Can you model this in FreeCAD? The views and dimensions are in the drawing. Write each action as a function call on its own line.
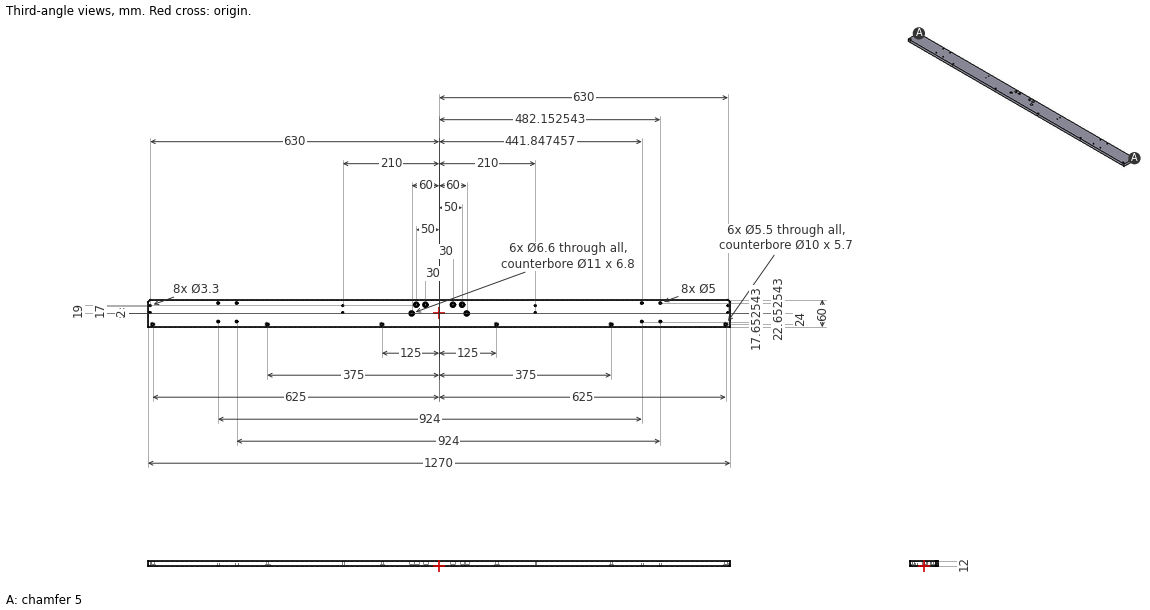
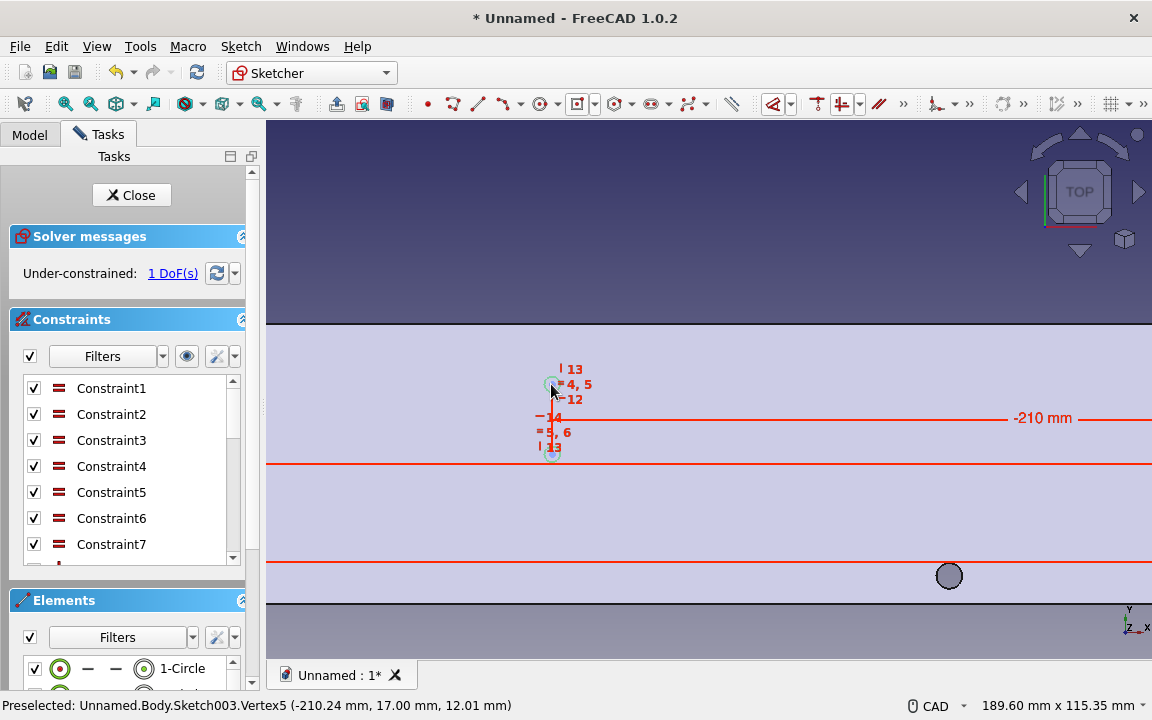
scroll(551, 386, down, 12)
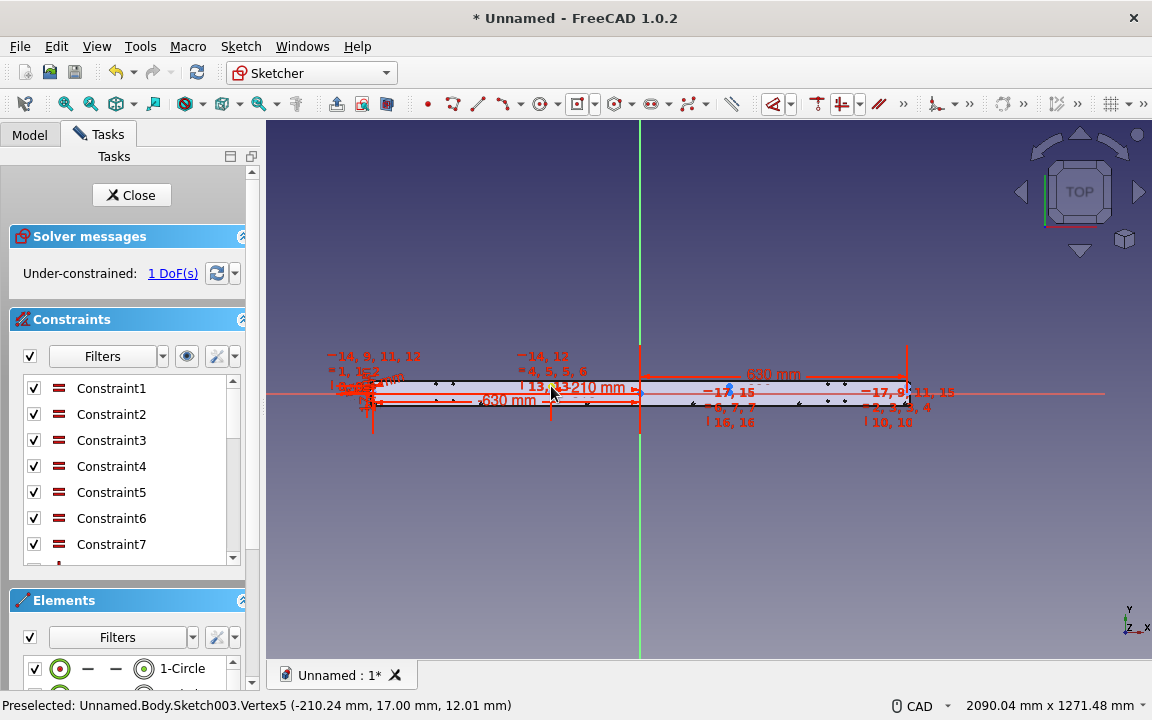
scroll(729, 393, up, 4)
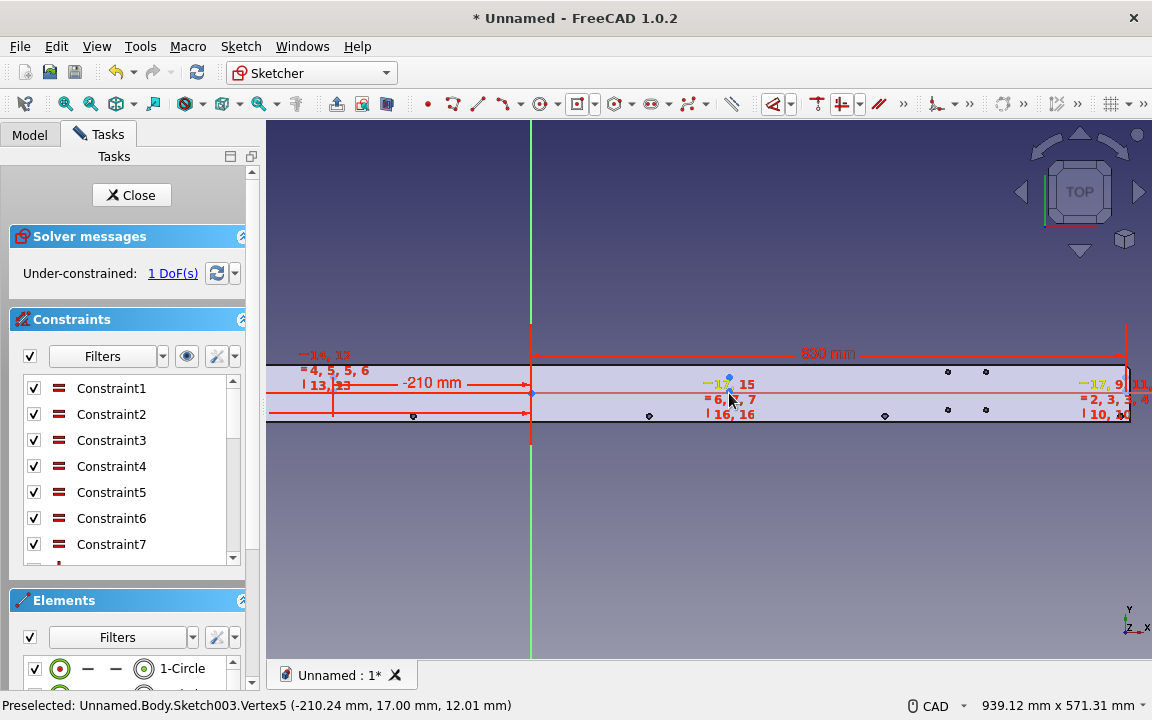
scroll(729, 392, up, 4)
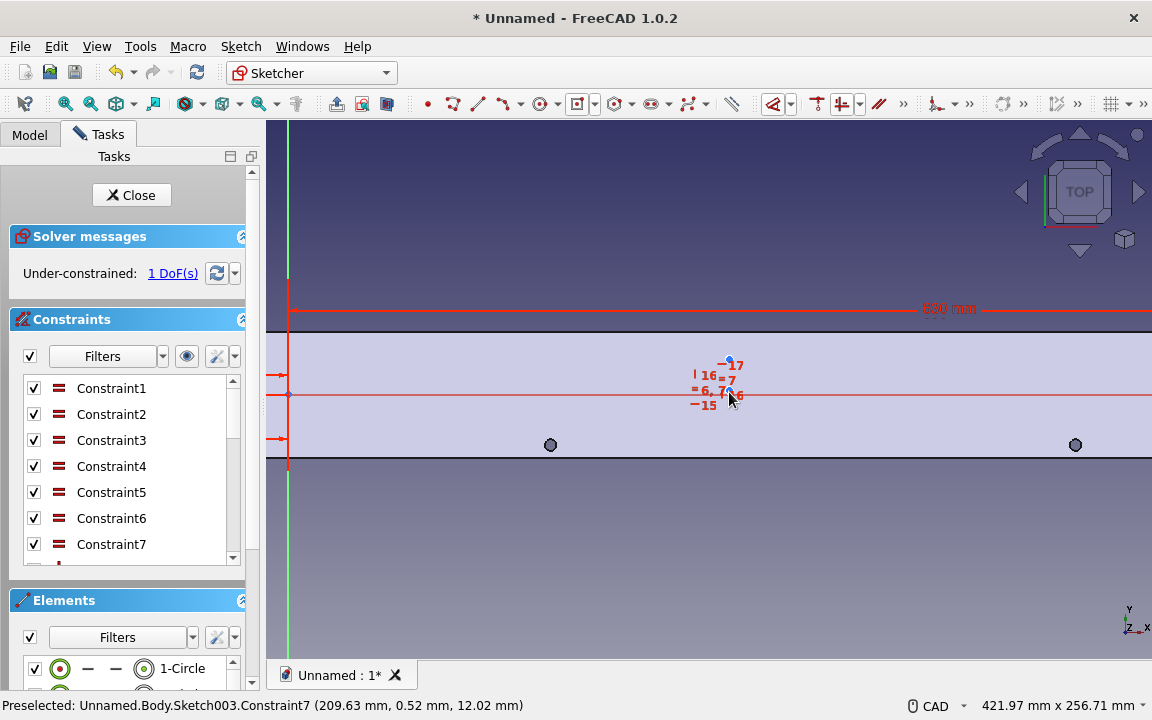
scroll(729, 391, up, 4)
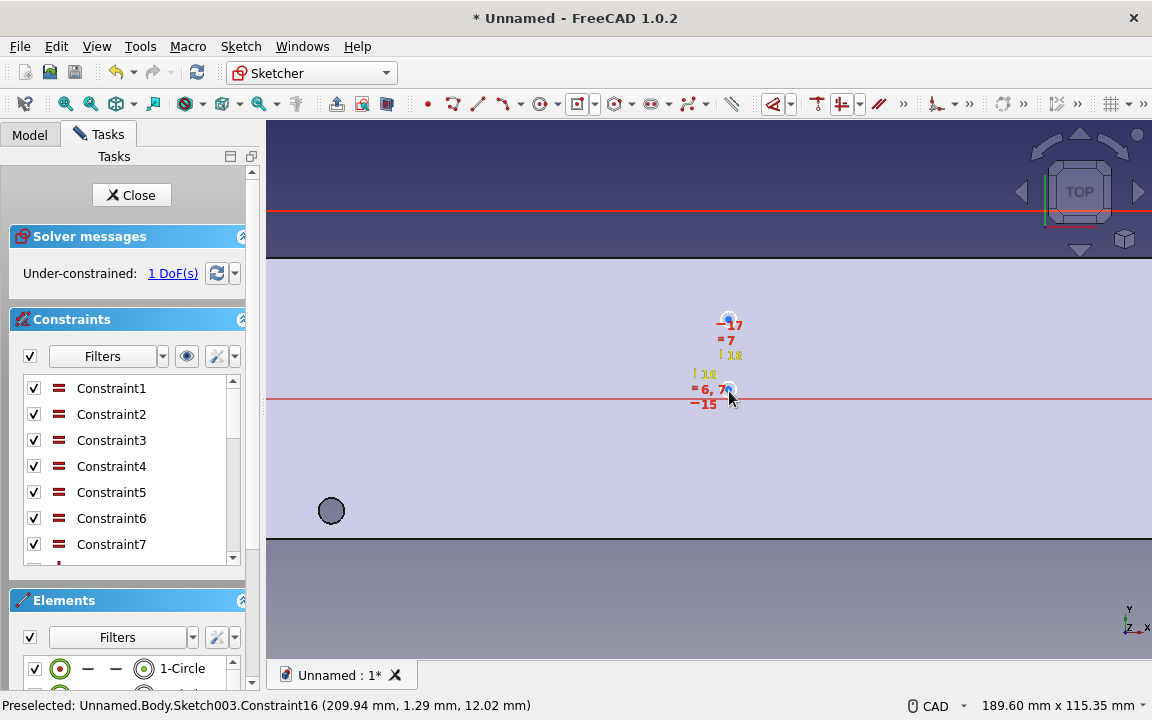
click(729, 389)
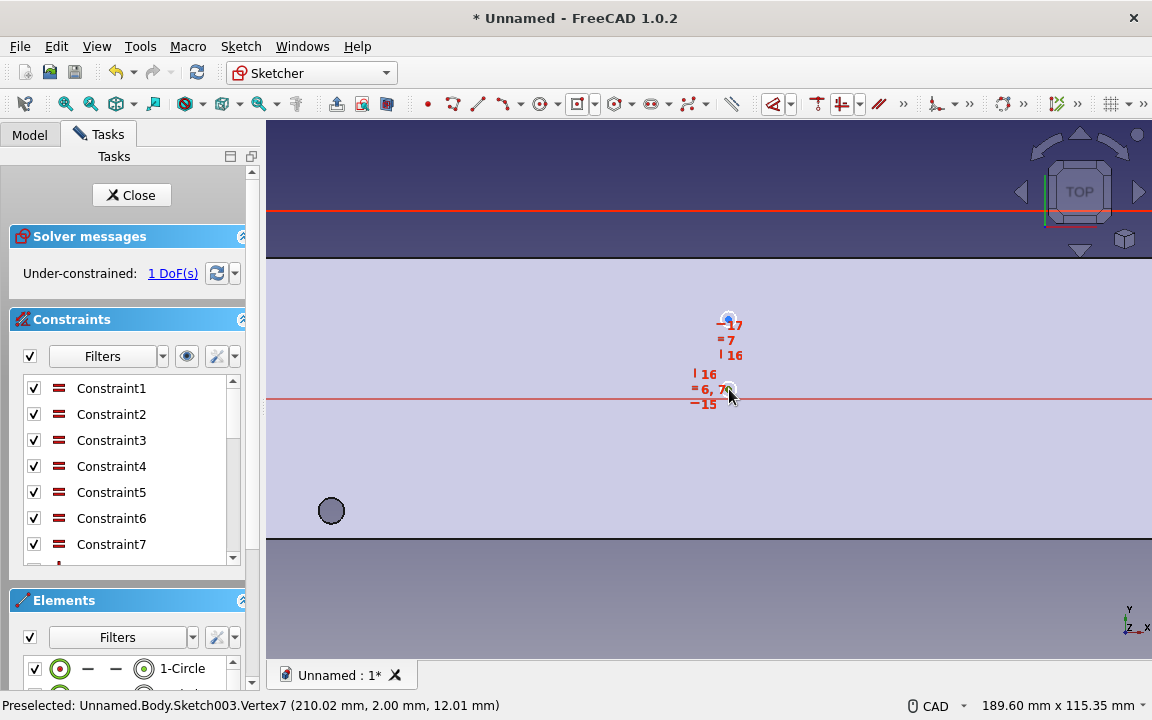
key(l)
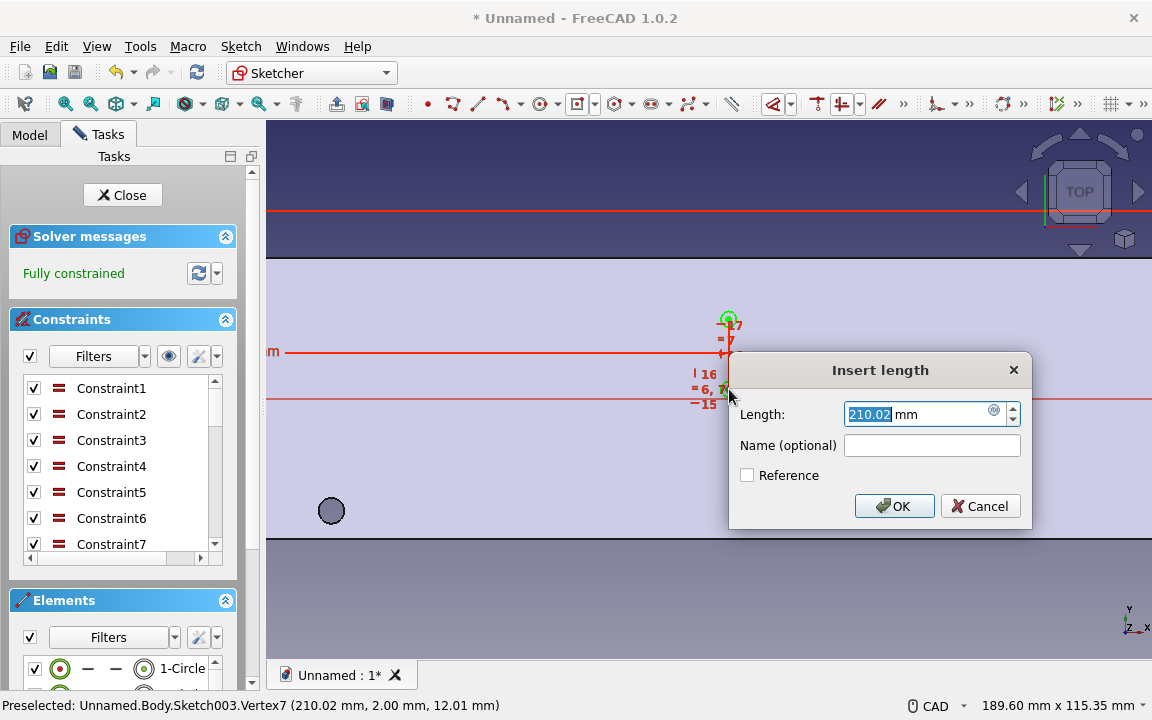
text(210)
key(Return)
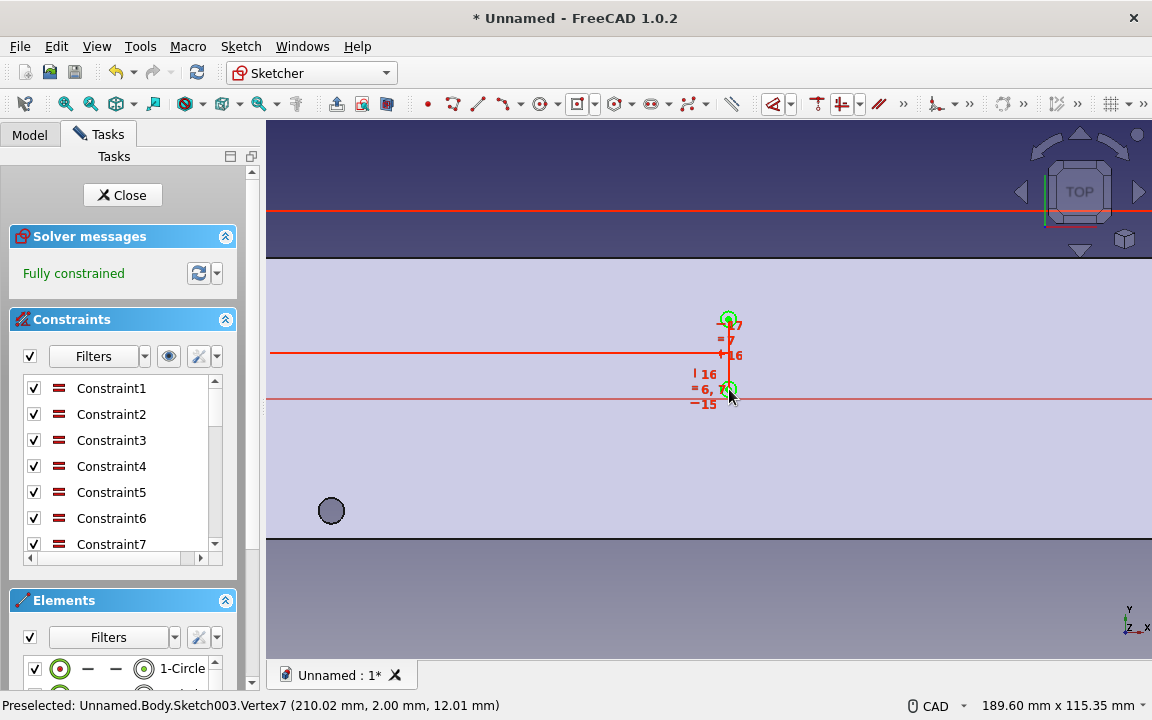
click(123, 195)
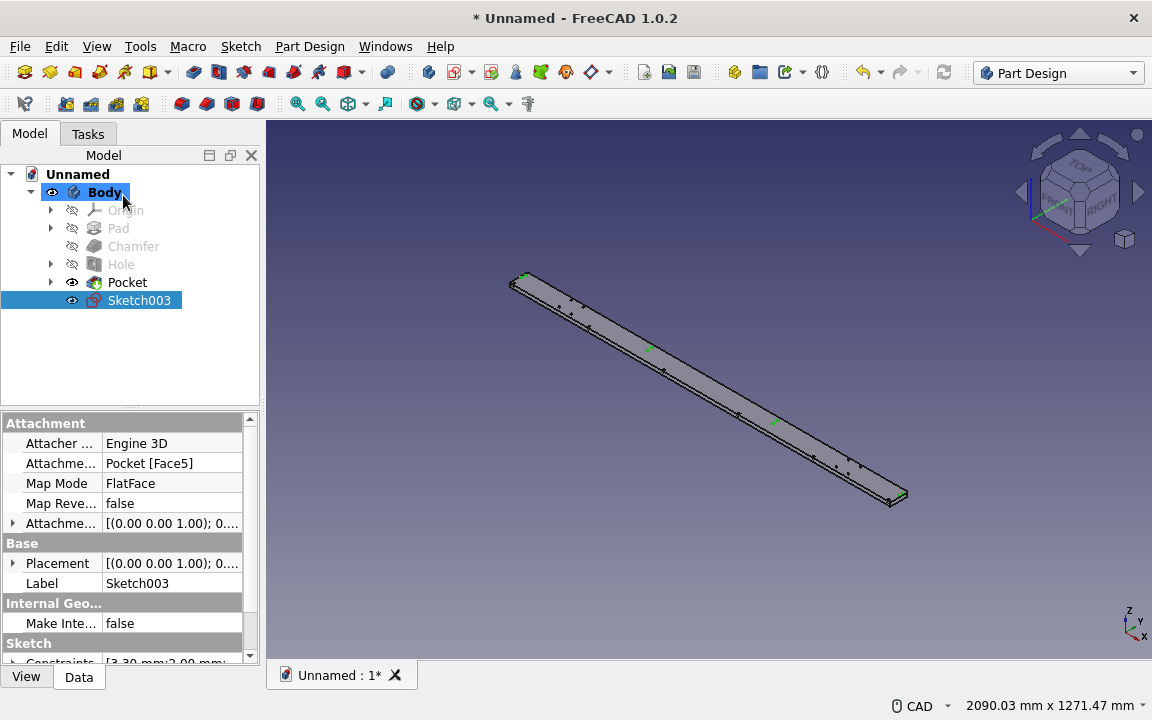
click(194, 72)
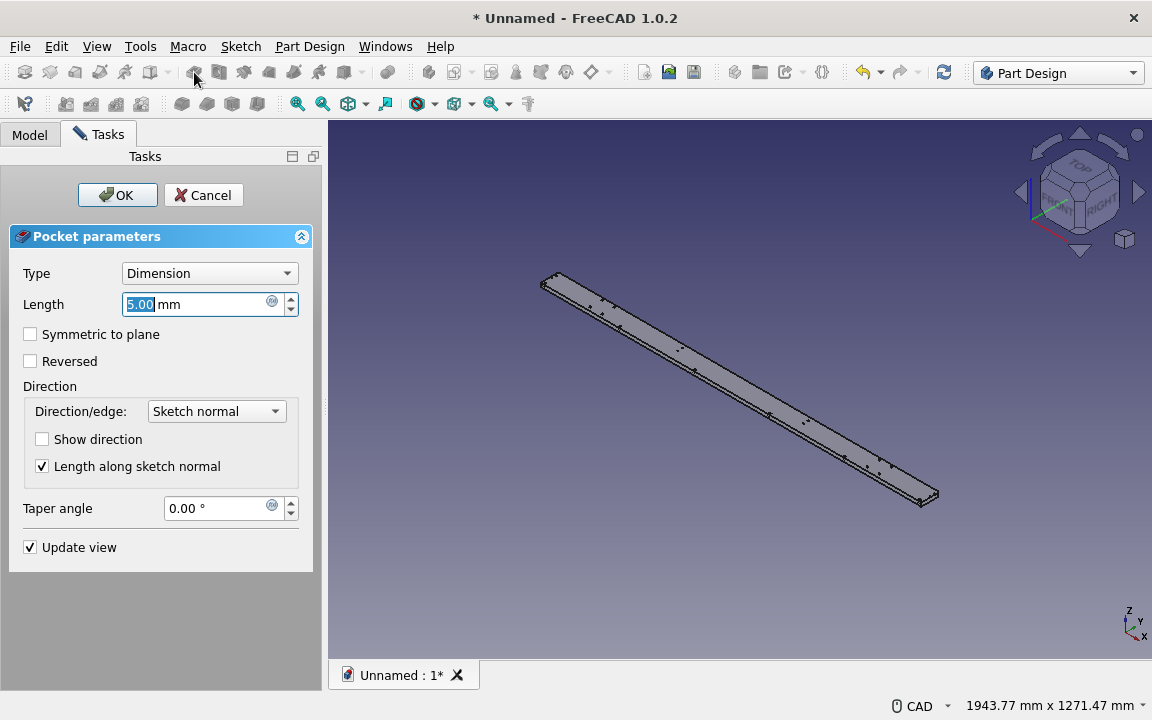
click(210, 274)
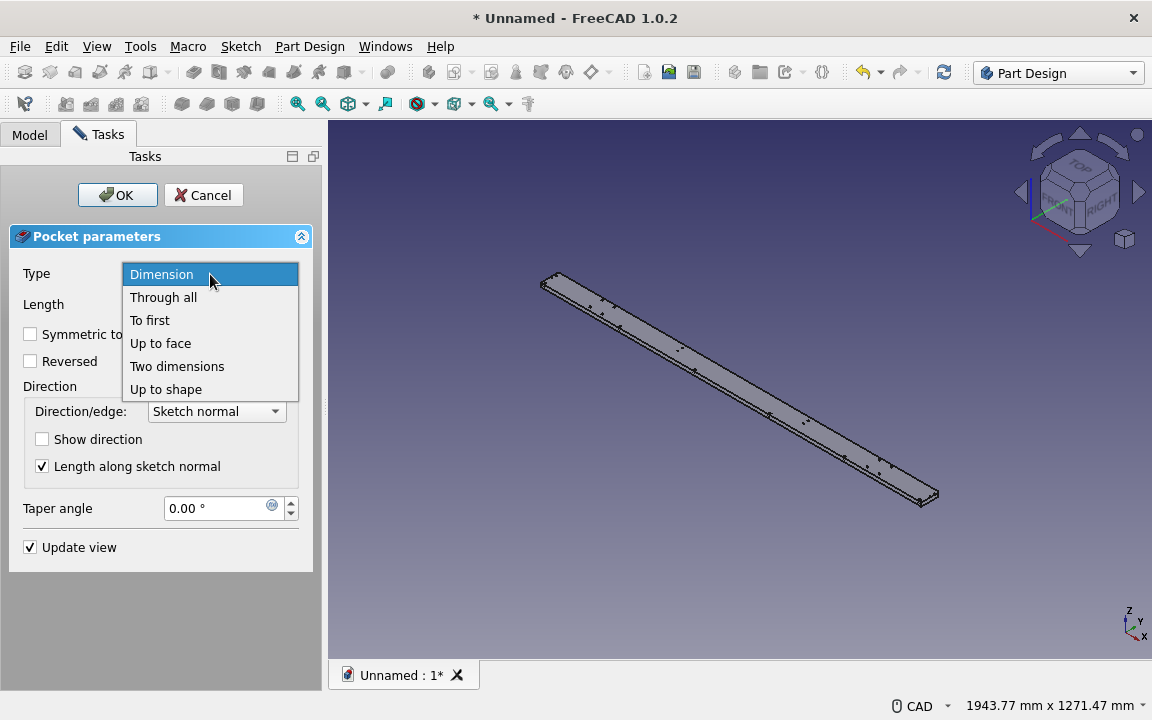
click(208, 298)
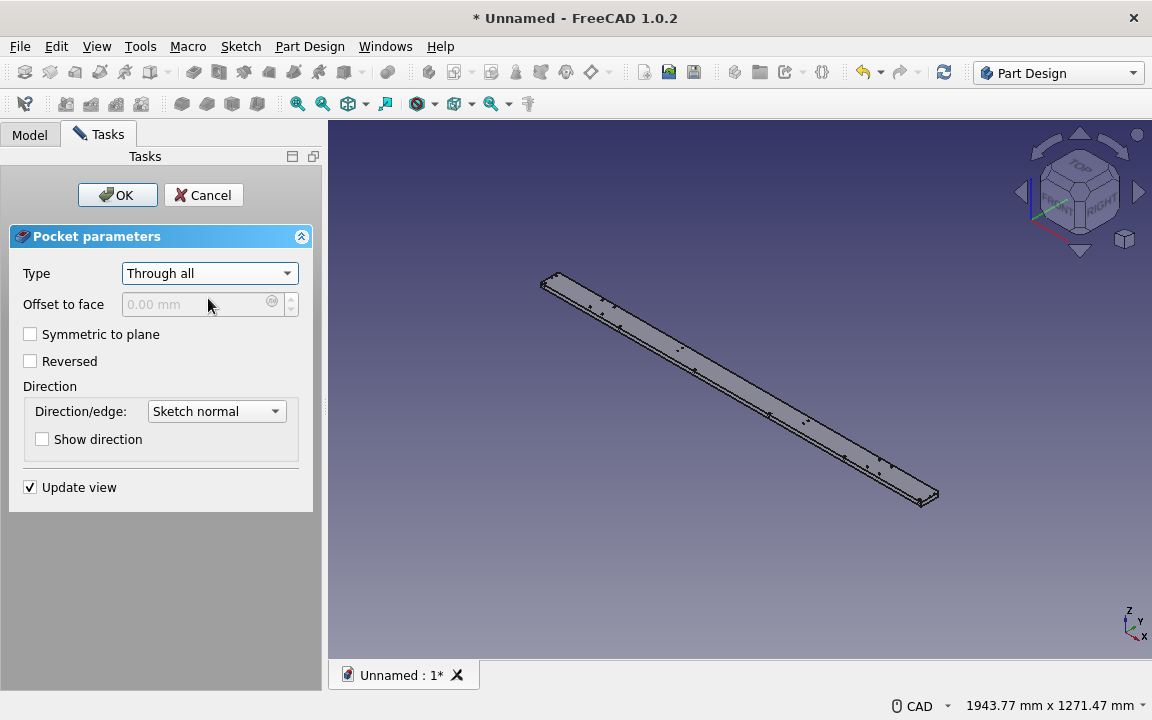
click(118, 195)